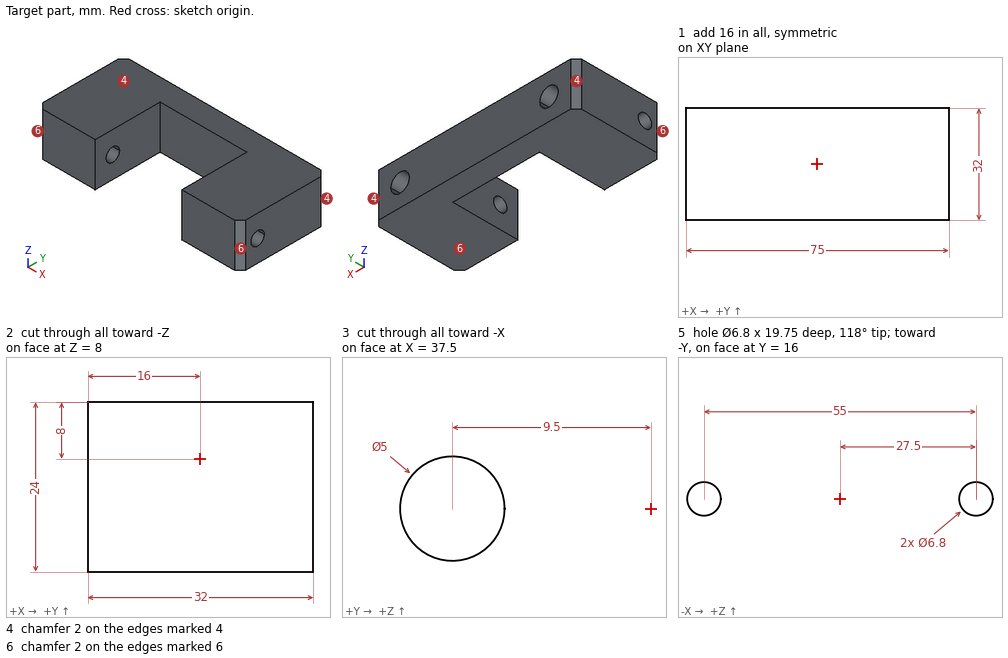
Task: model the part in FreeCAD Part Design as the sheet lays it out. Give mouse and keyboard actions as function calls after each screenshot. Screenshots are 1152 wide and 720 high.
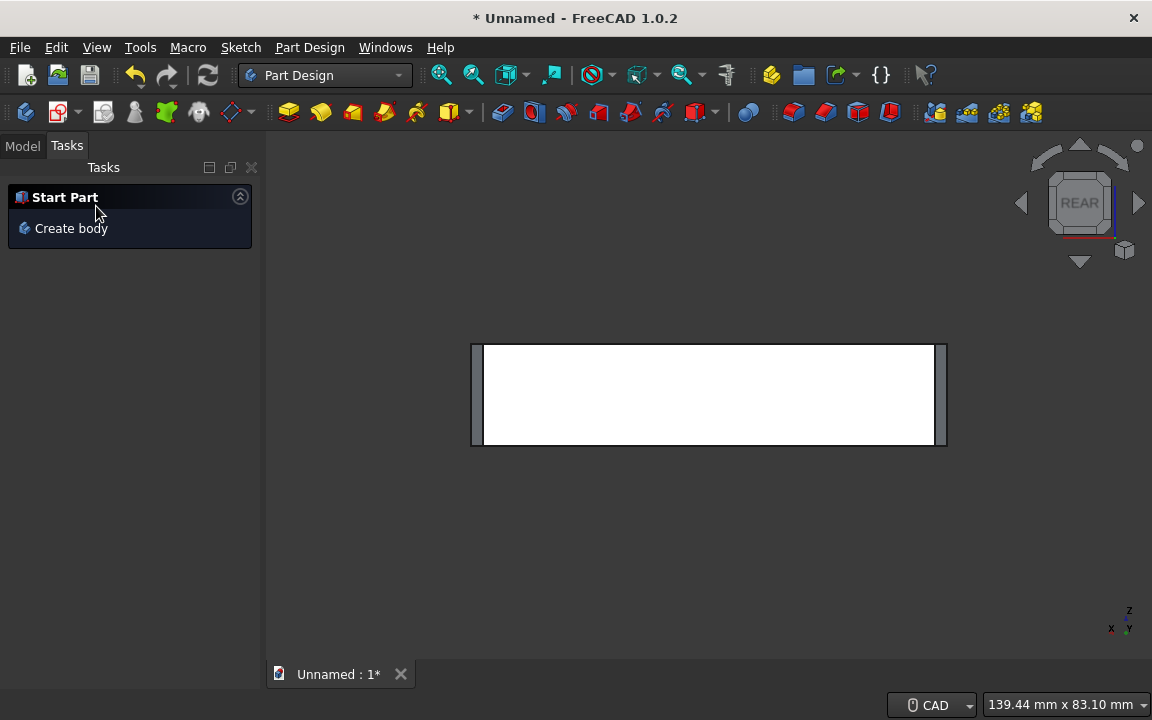
click(580, 394)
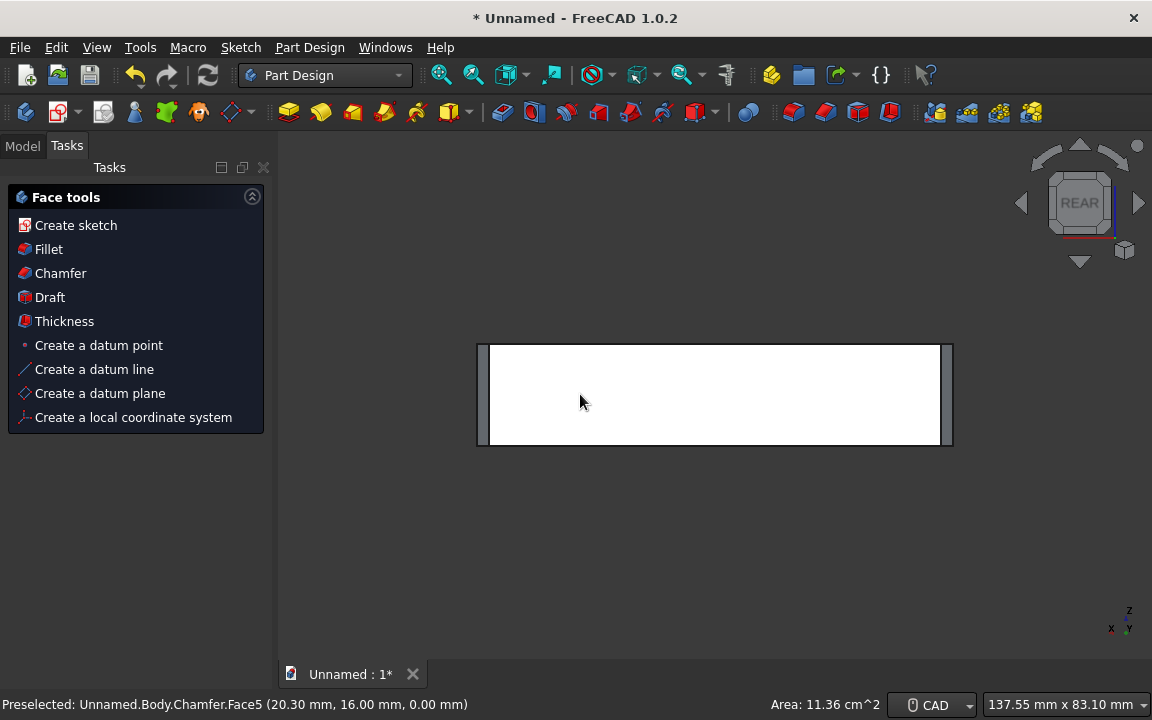
click(58, 112)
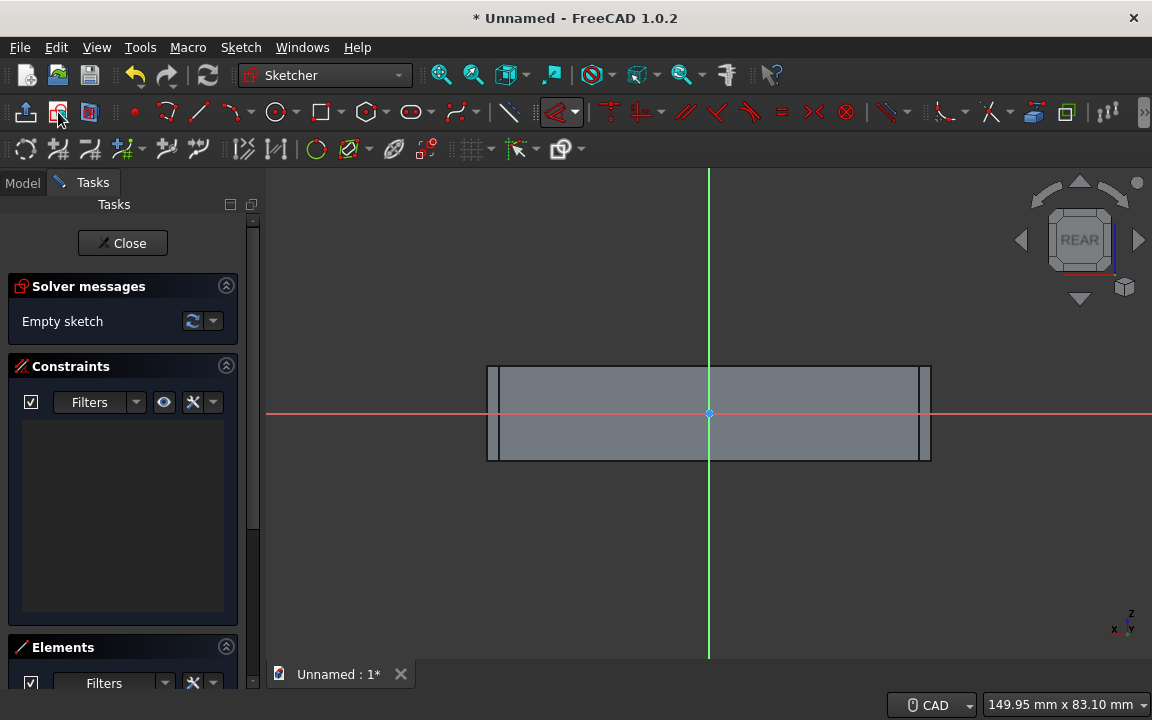
key(g)
key(c)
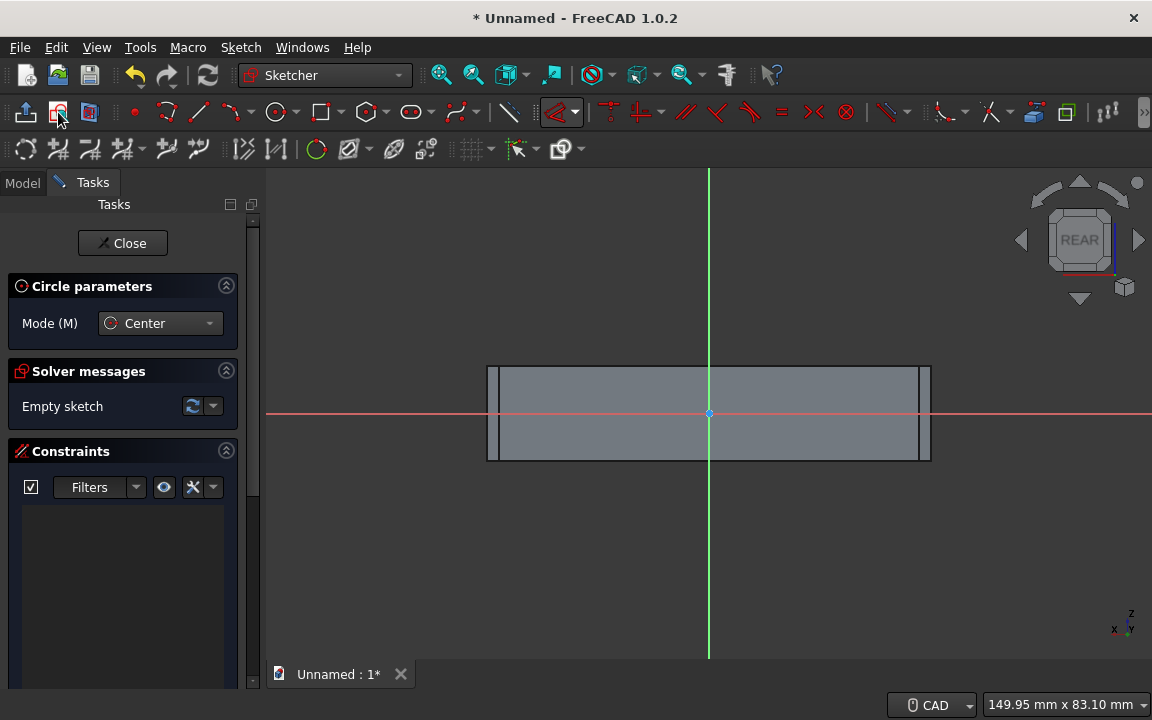
click(871, 413)
click(886, 399)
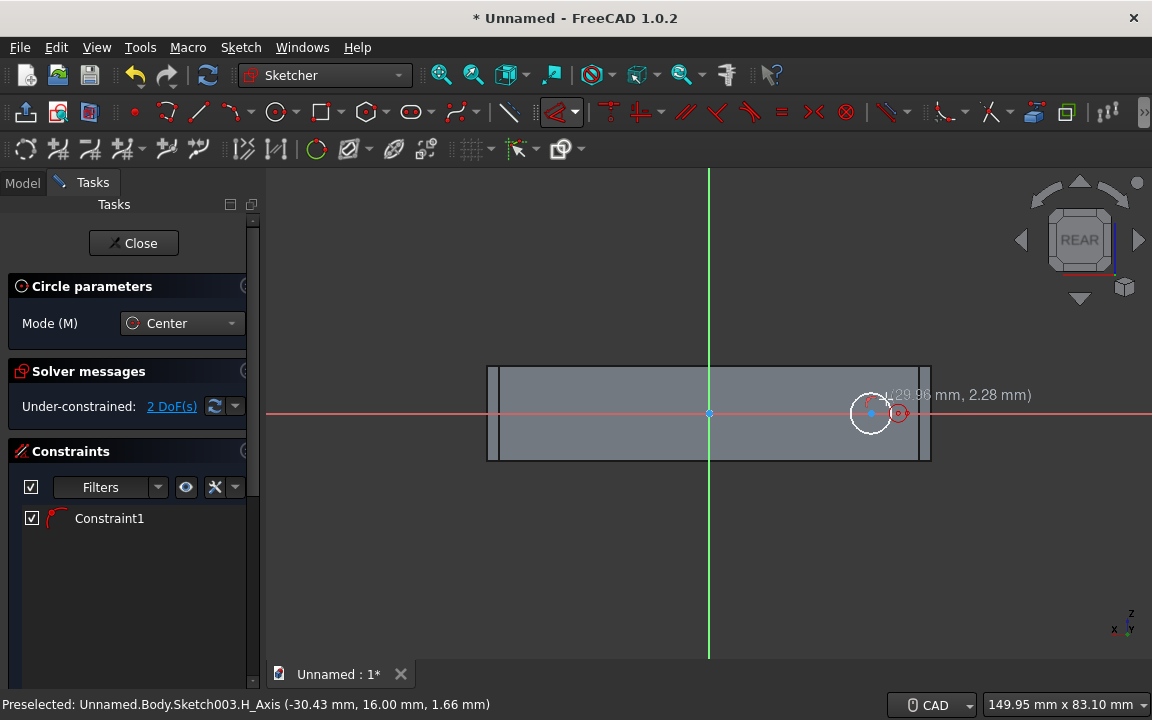
click(547, 413)
click(561, 399)
key(Escape)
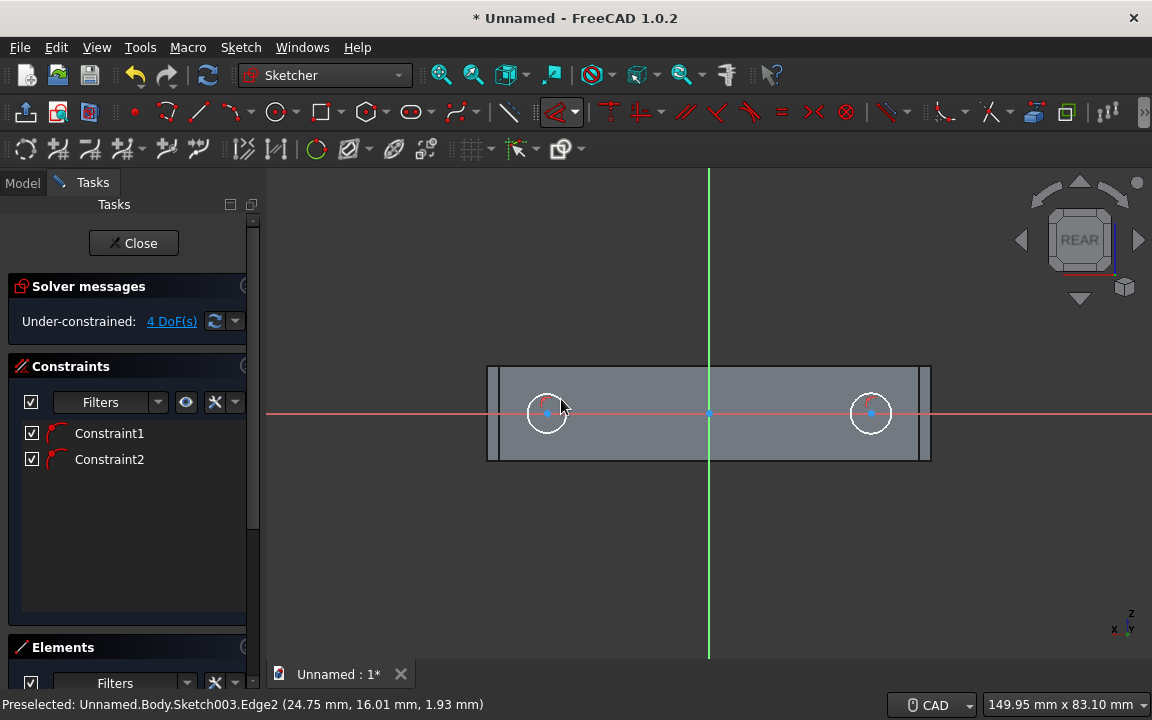
click(885, 399)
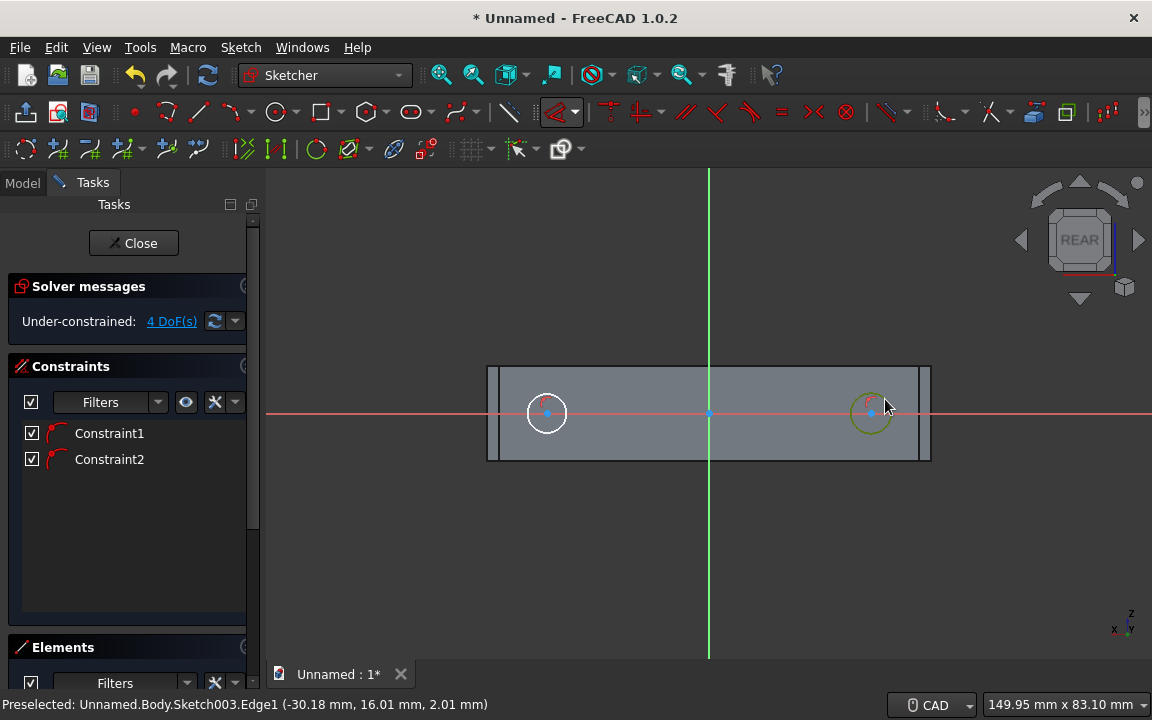
click(561, 400)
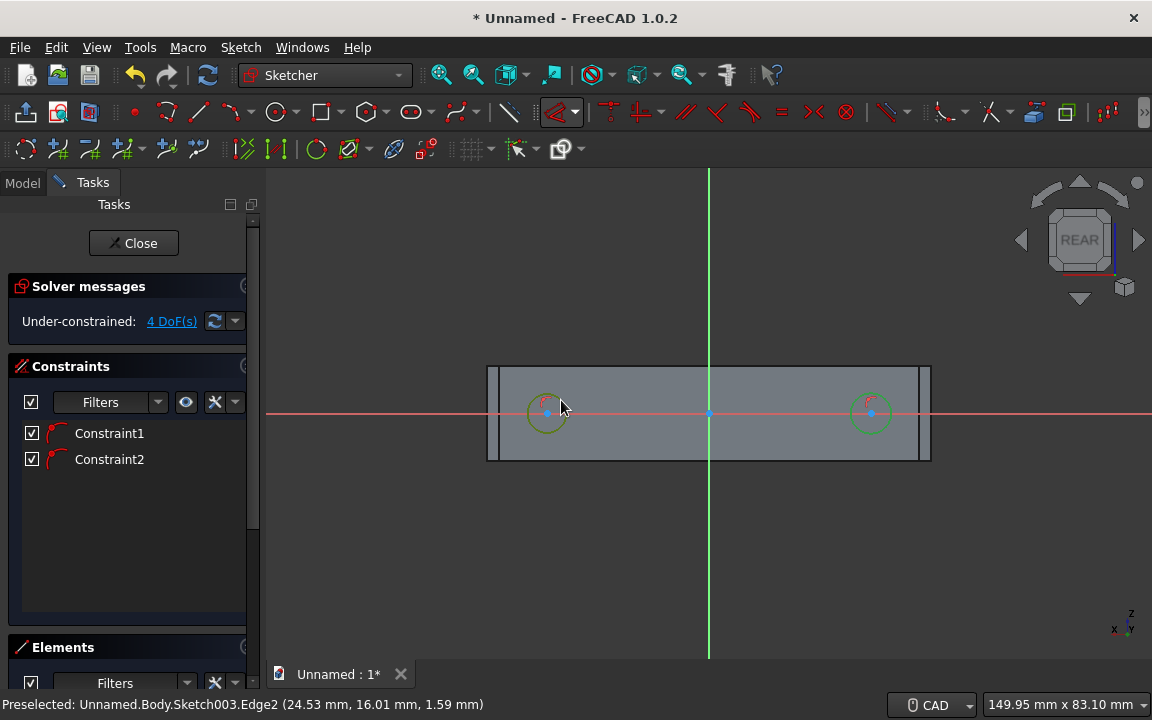
key(e)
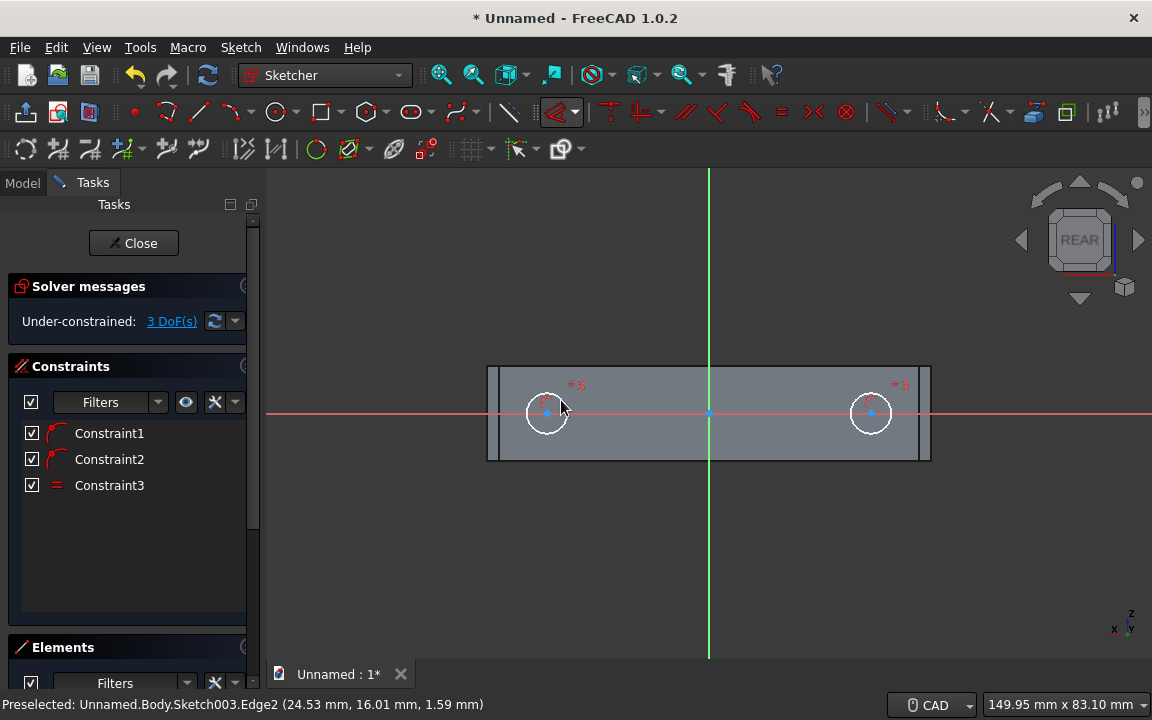
click(885, 399)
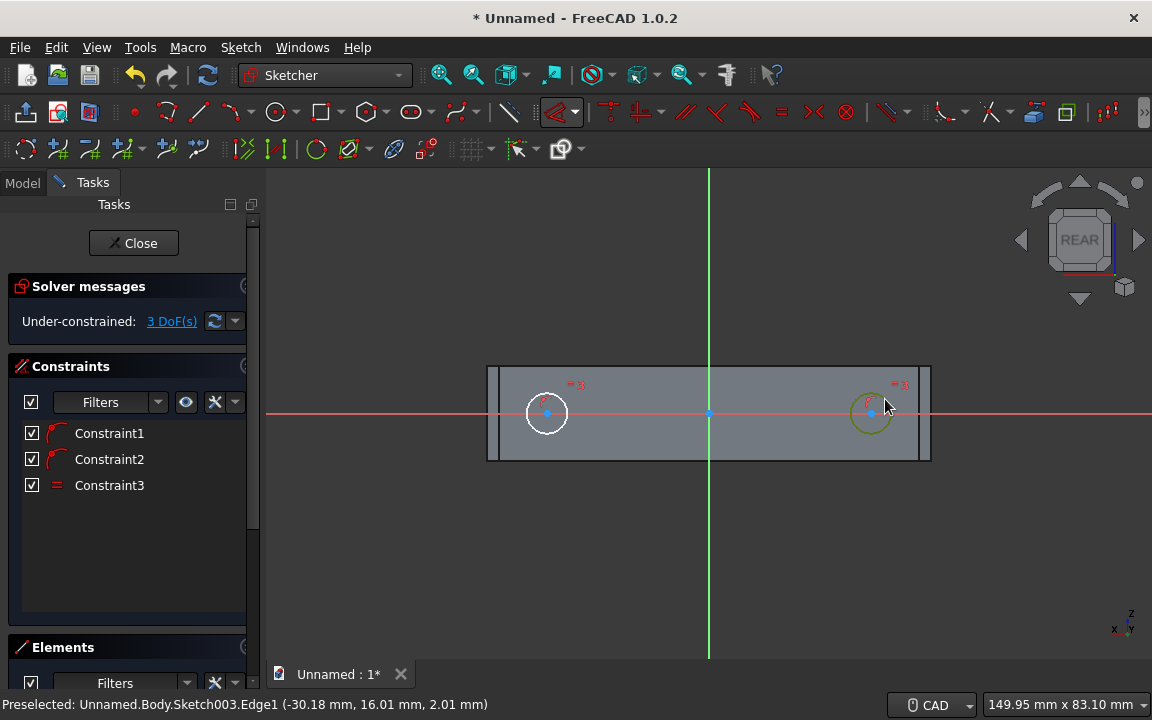
key(k)
key(o)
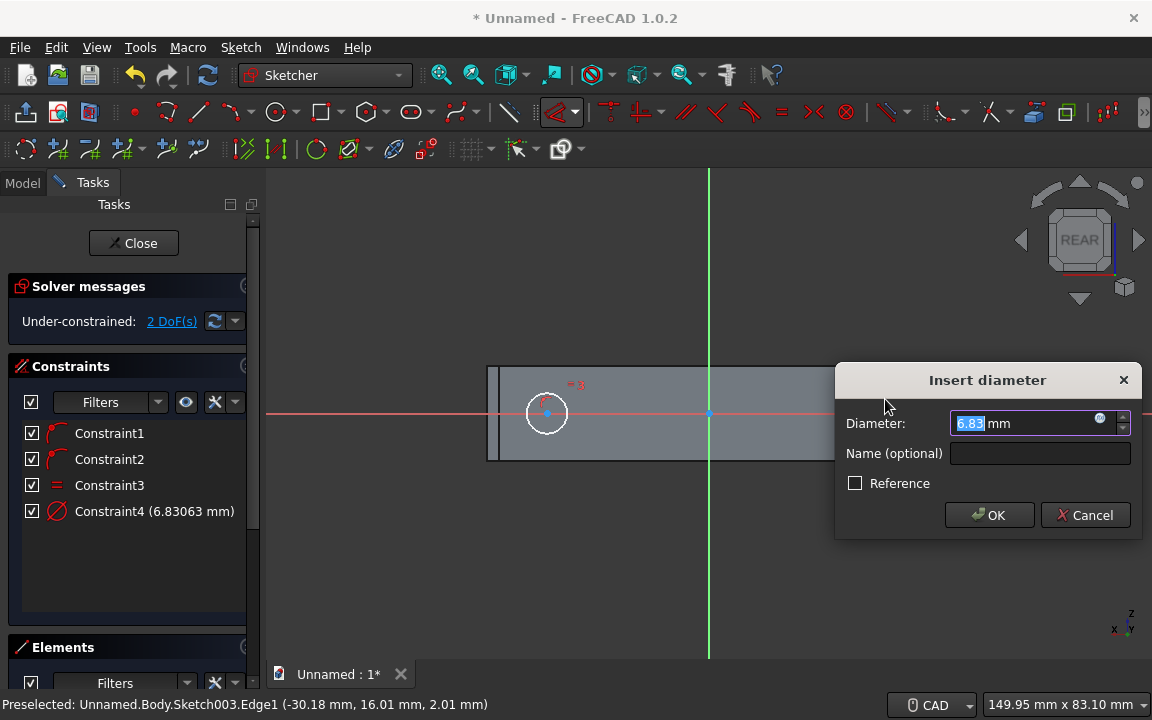
text(6.8)
key(Return)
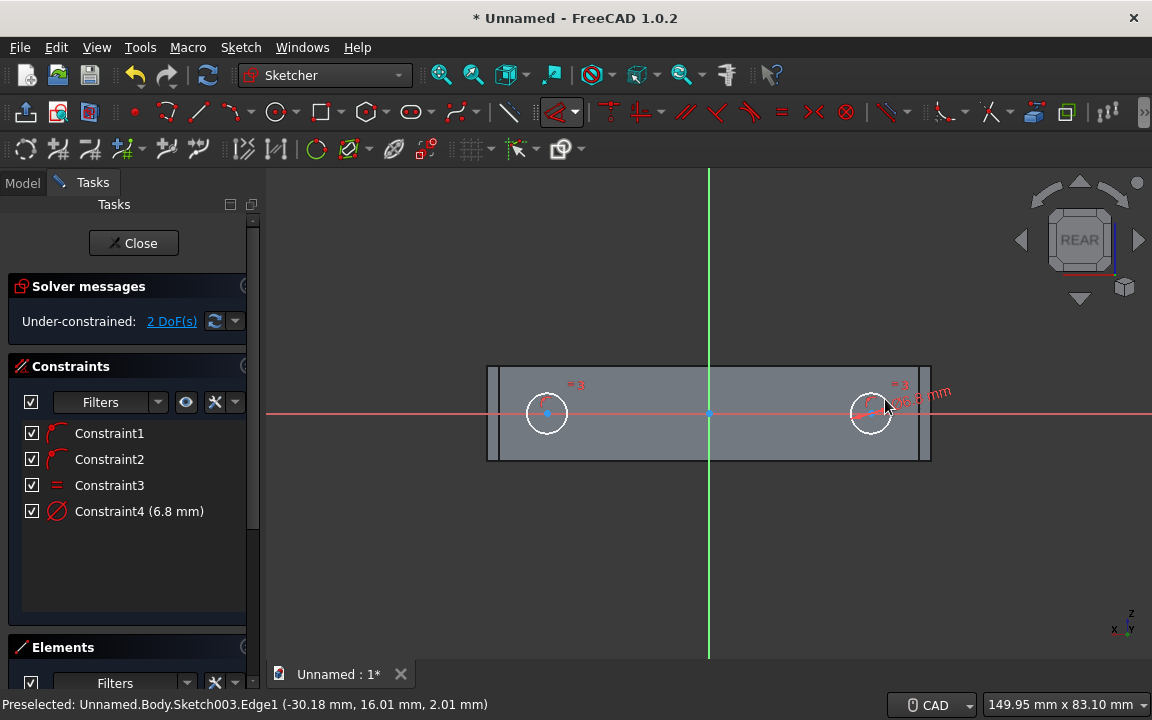
click(871, 413)